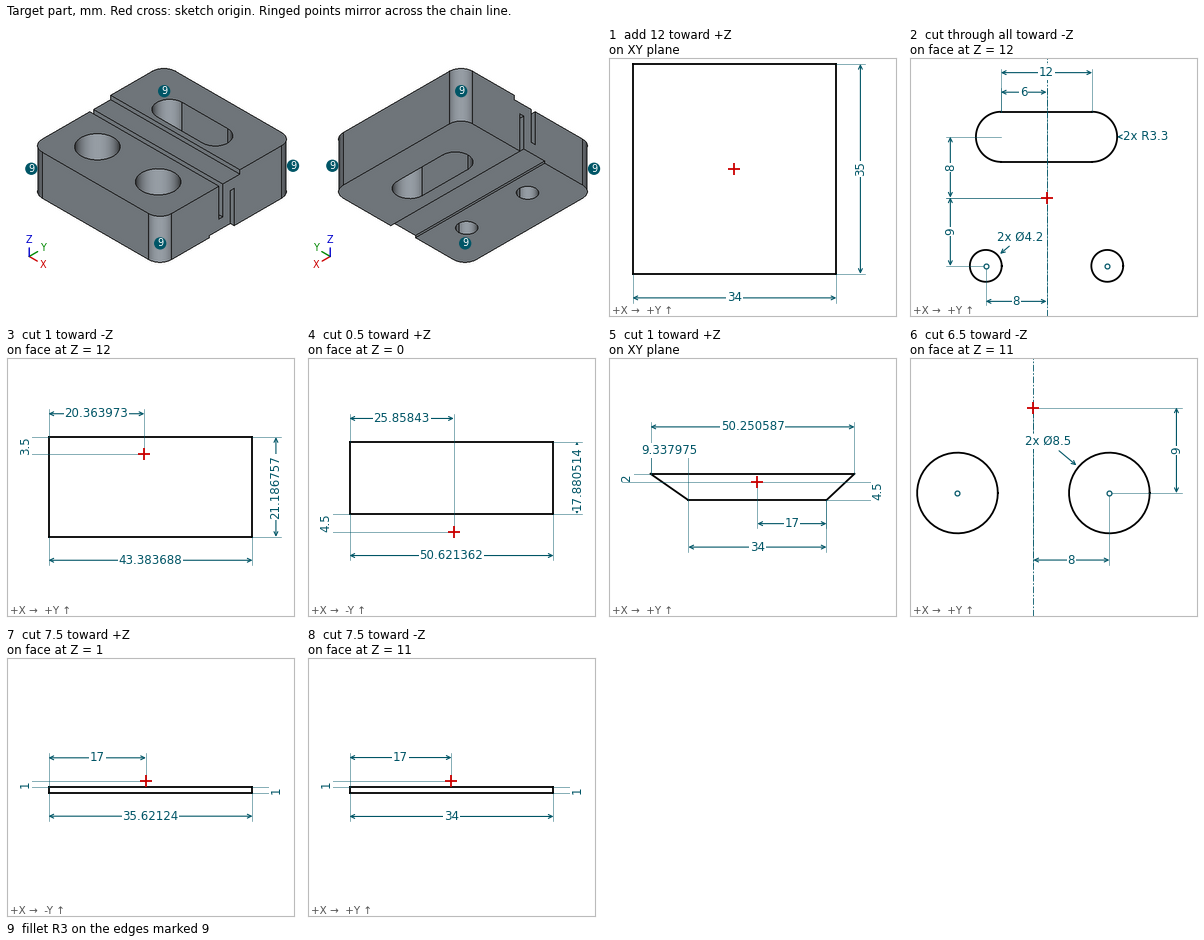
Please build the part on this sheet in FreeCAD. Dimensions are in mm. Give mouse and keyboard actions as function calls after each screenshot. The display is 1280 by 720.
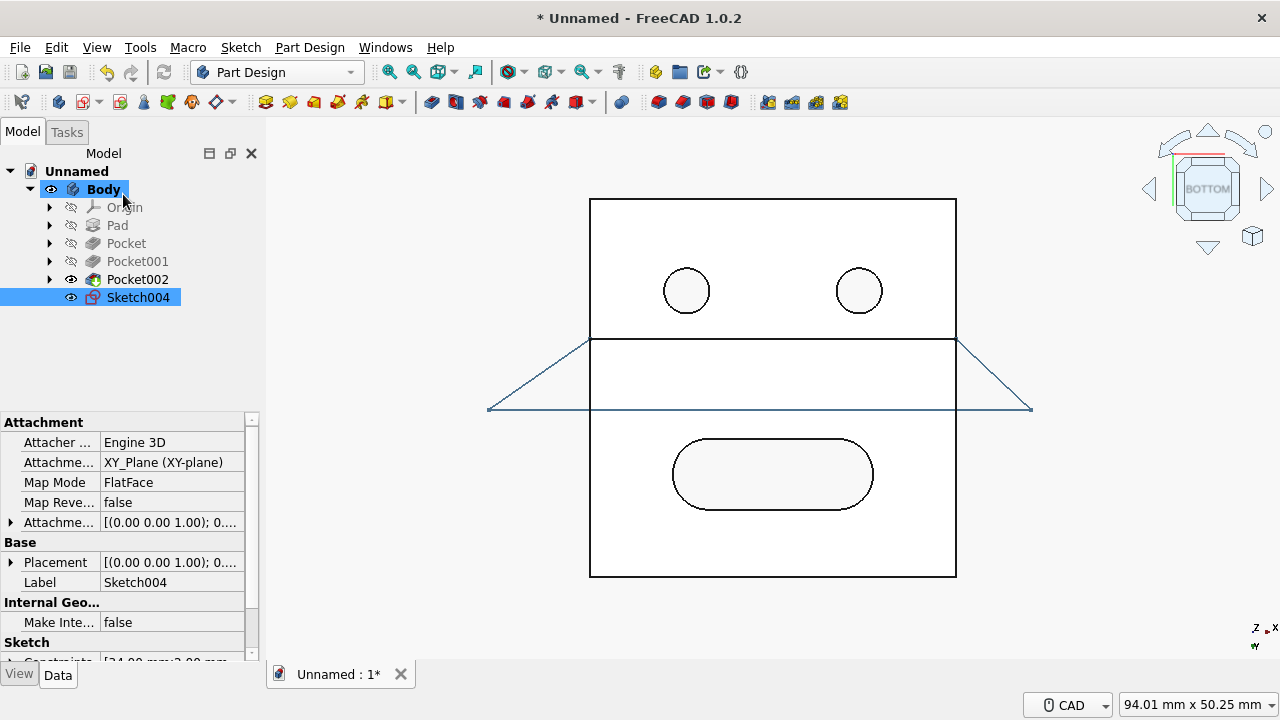
click(432, 102)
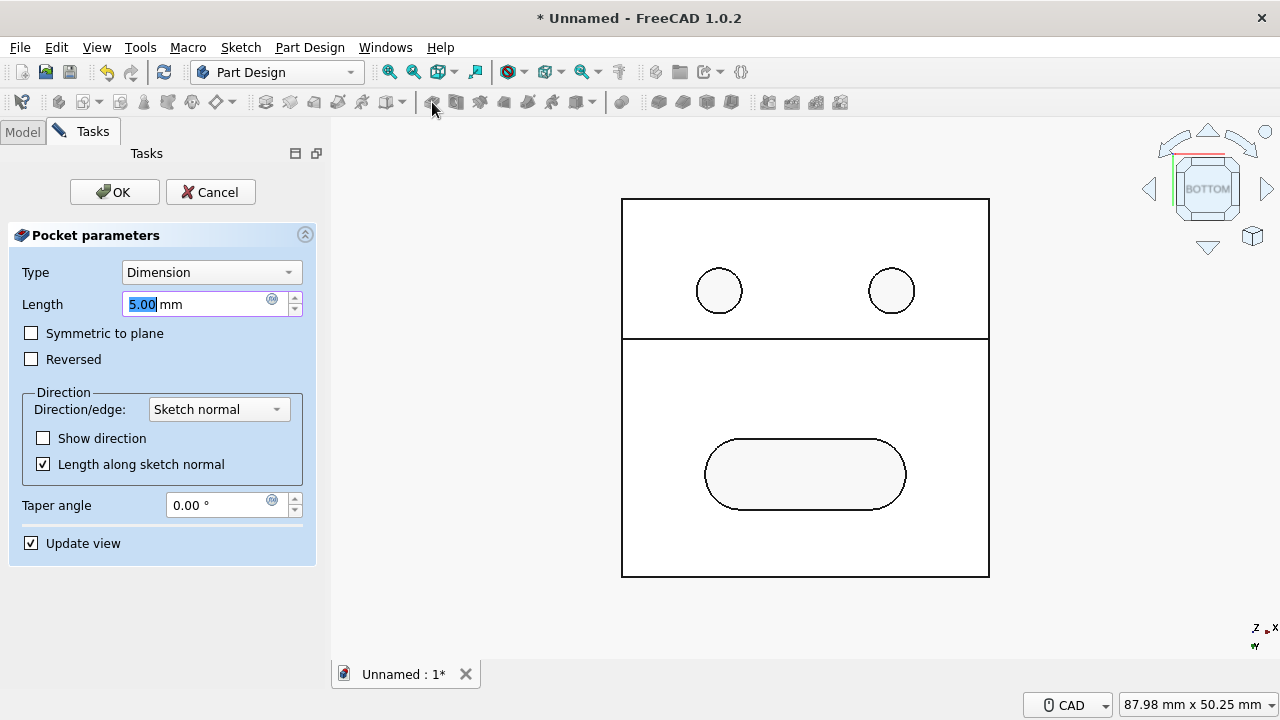
text(1)
key(Tab)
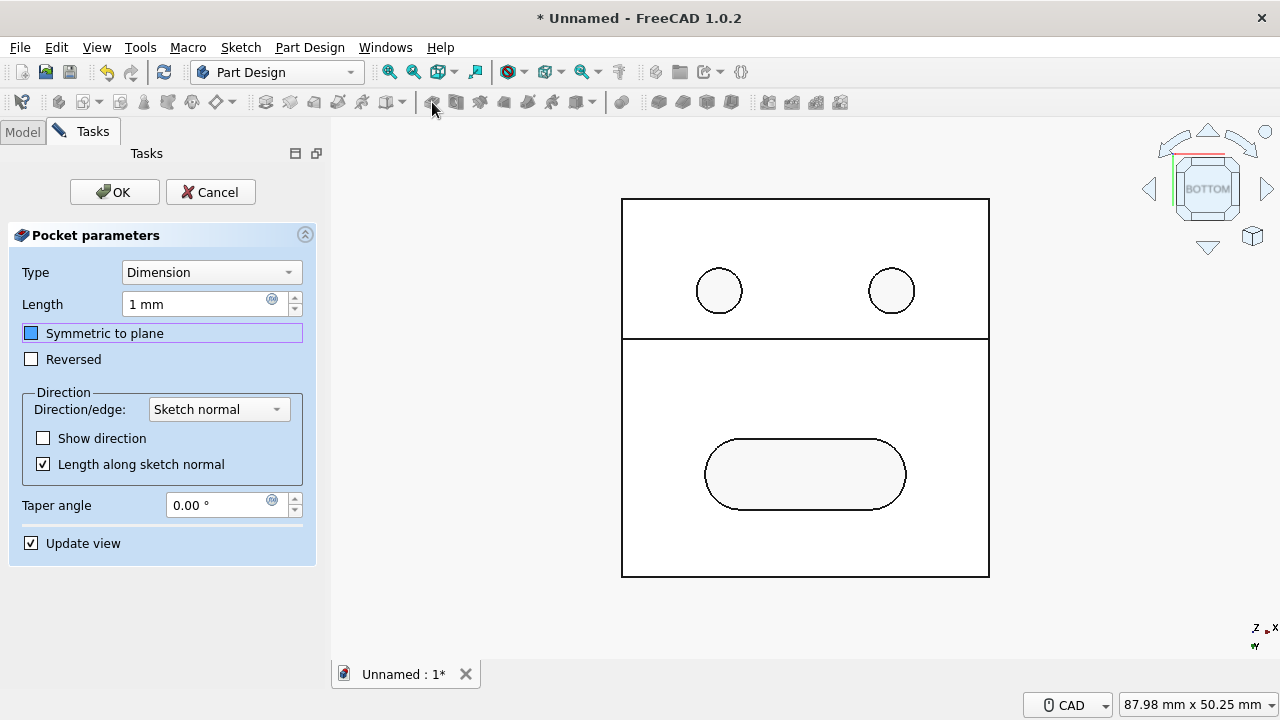
click(30, 359)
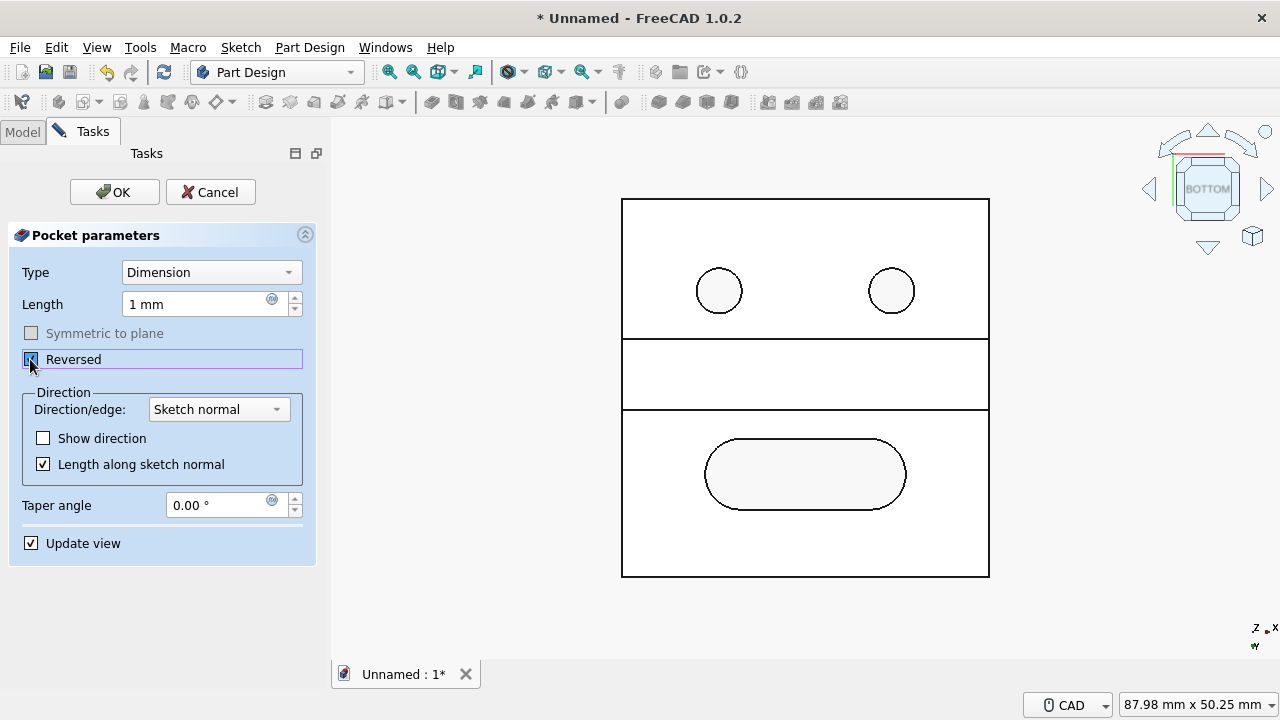
click(115, 192)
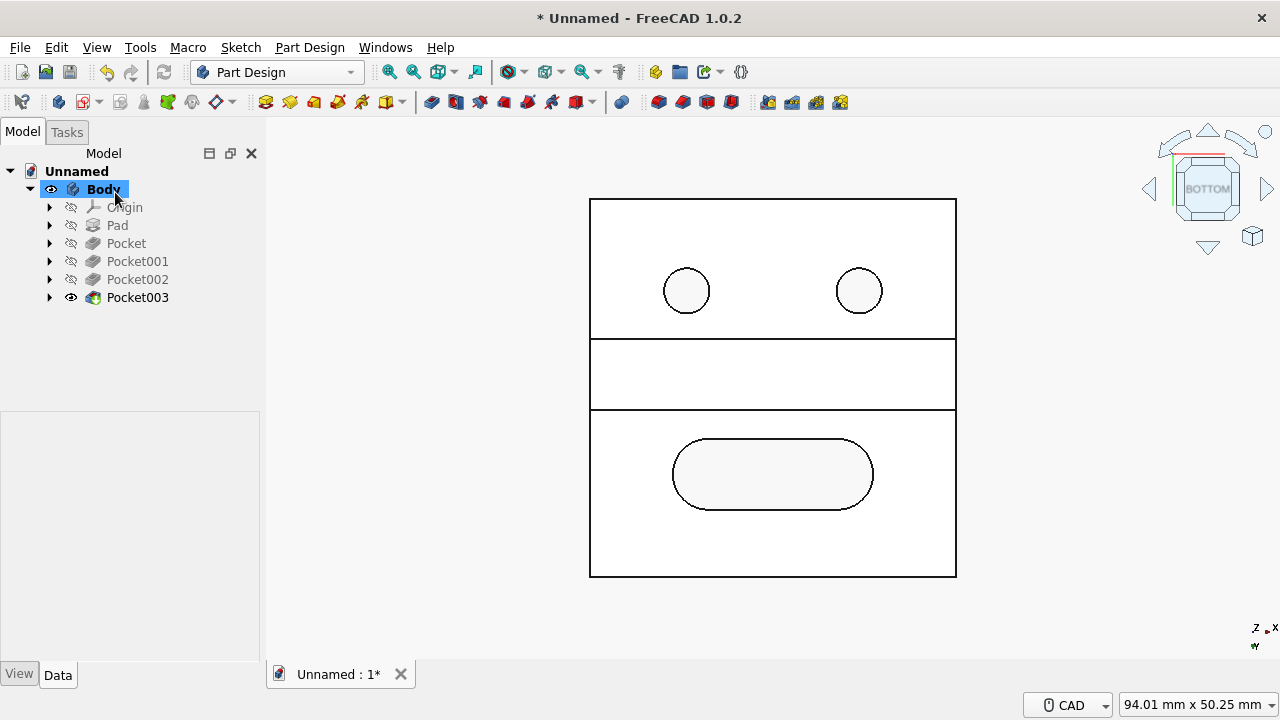
key(0)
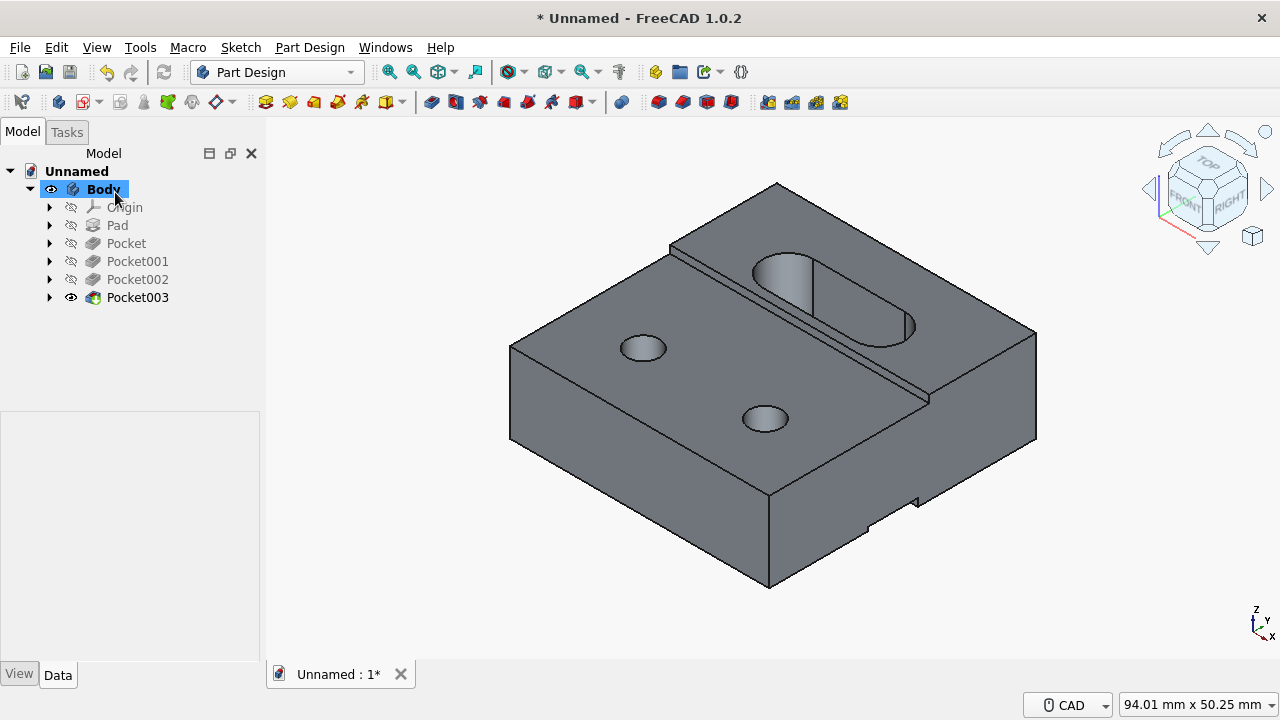
click(742, 361)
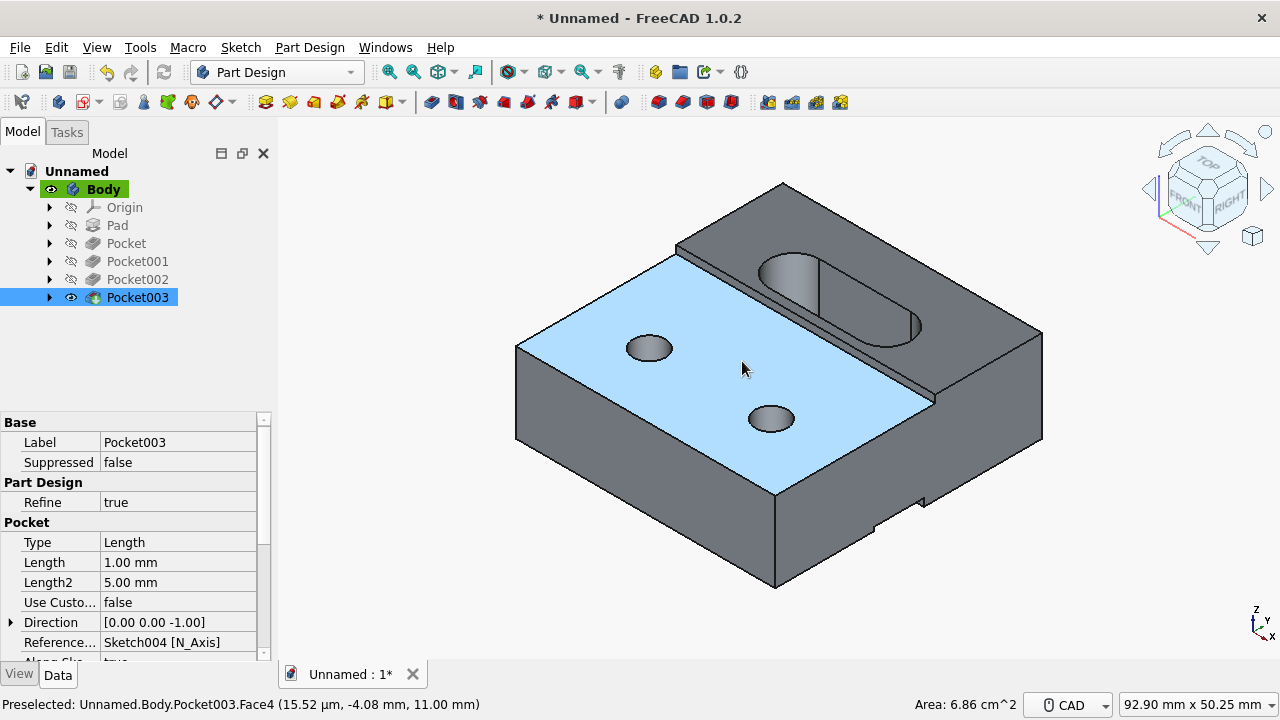
click(84, 102)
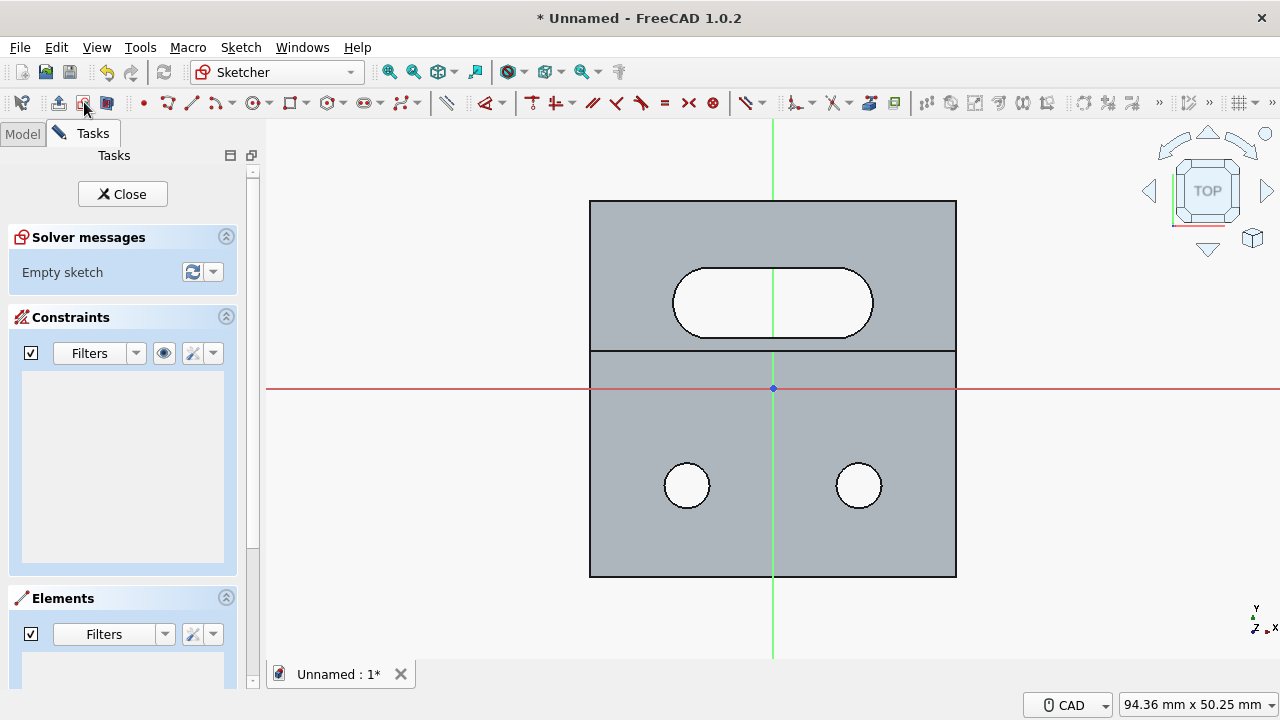
scroll(829, 518, up, 4)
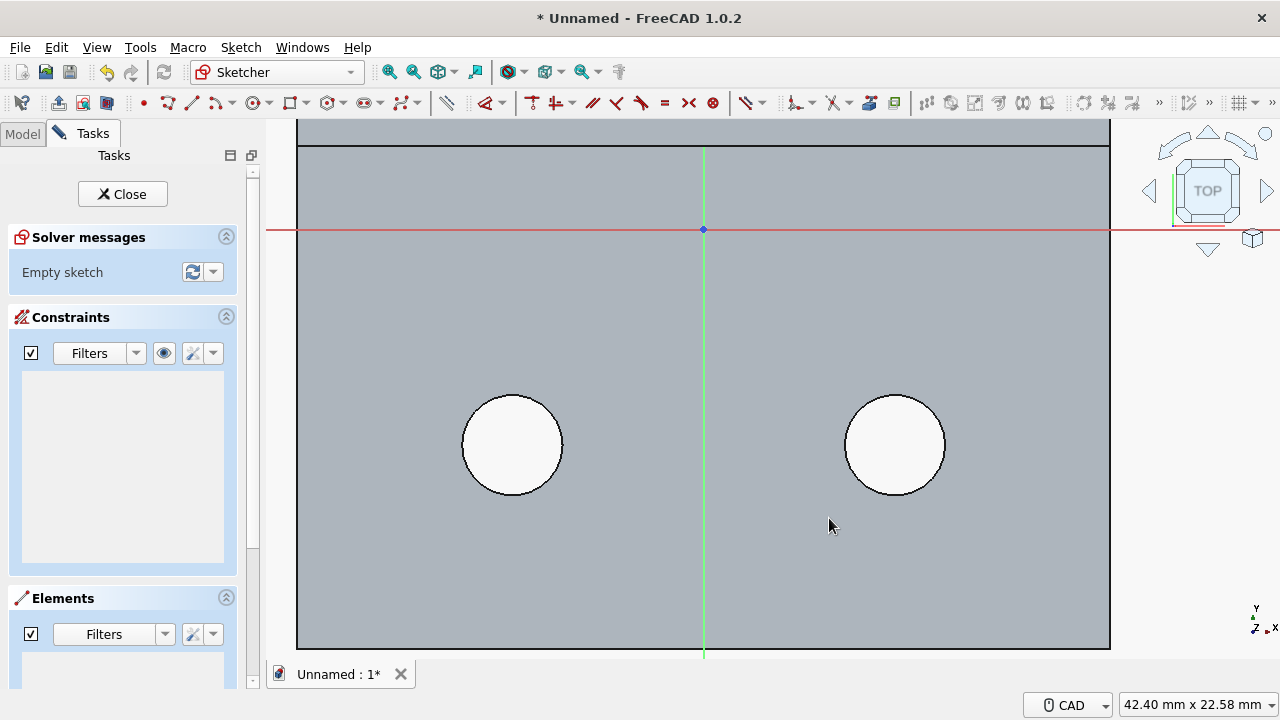
key(g)
key(c)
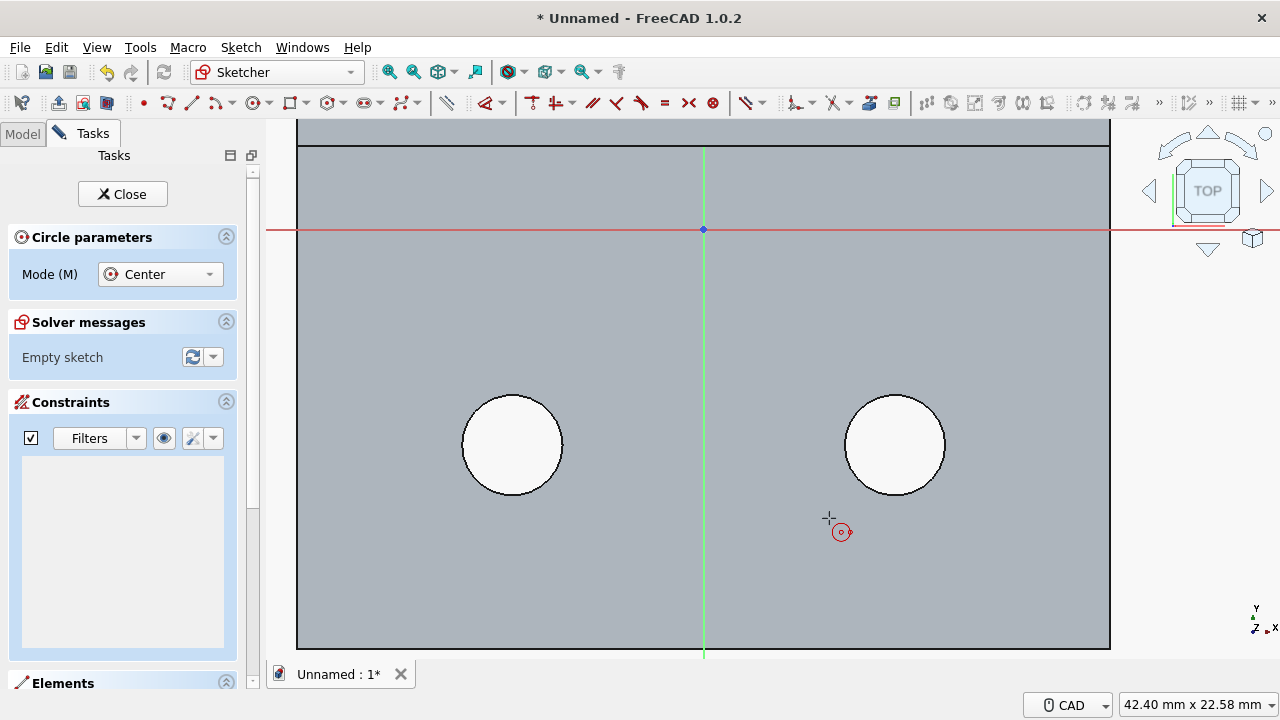
click(895, 445)
move(967, 373)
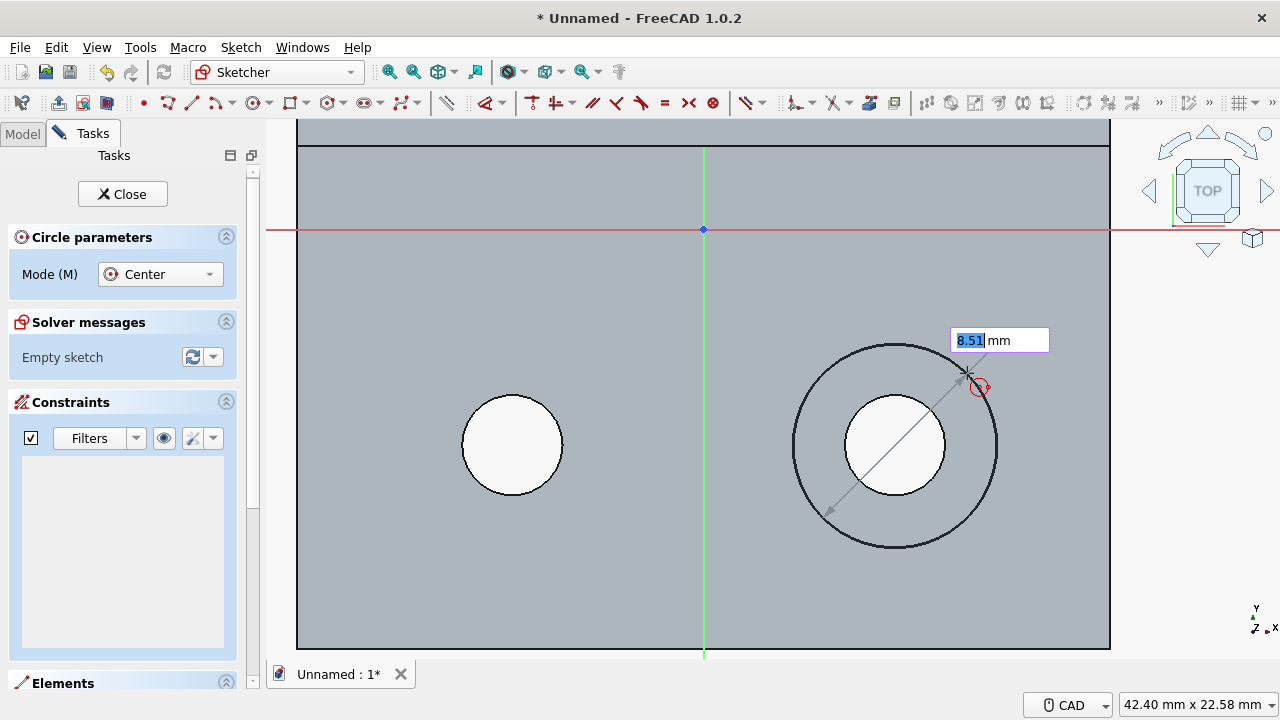
text(8.5)
key(Return)